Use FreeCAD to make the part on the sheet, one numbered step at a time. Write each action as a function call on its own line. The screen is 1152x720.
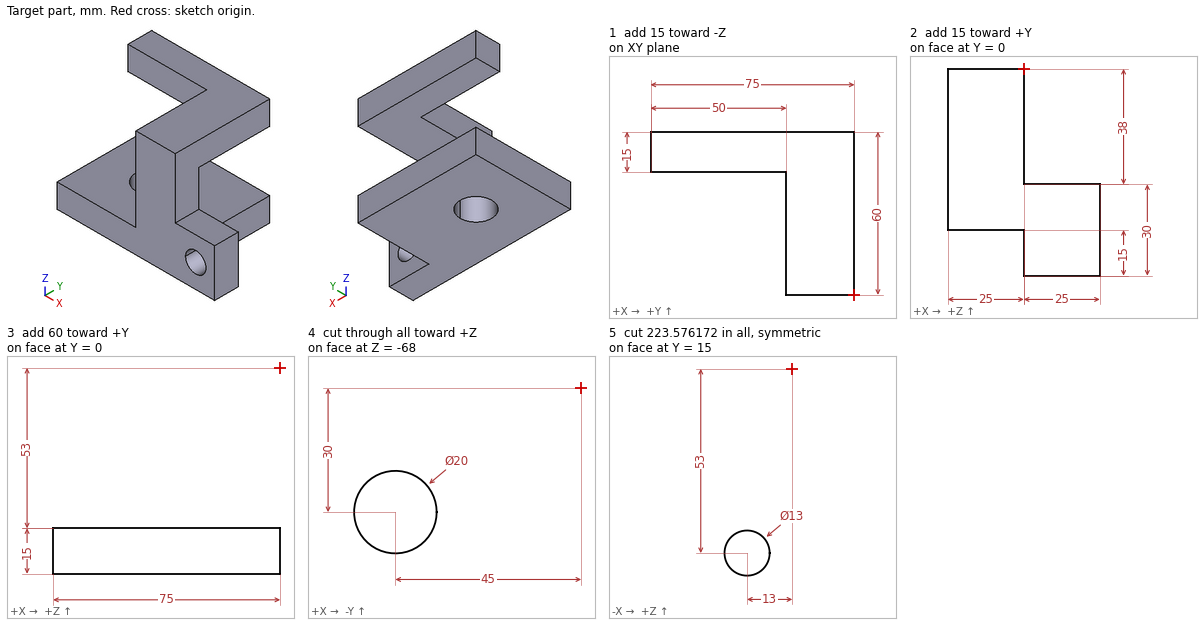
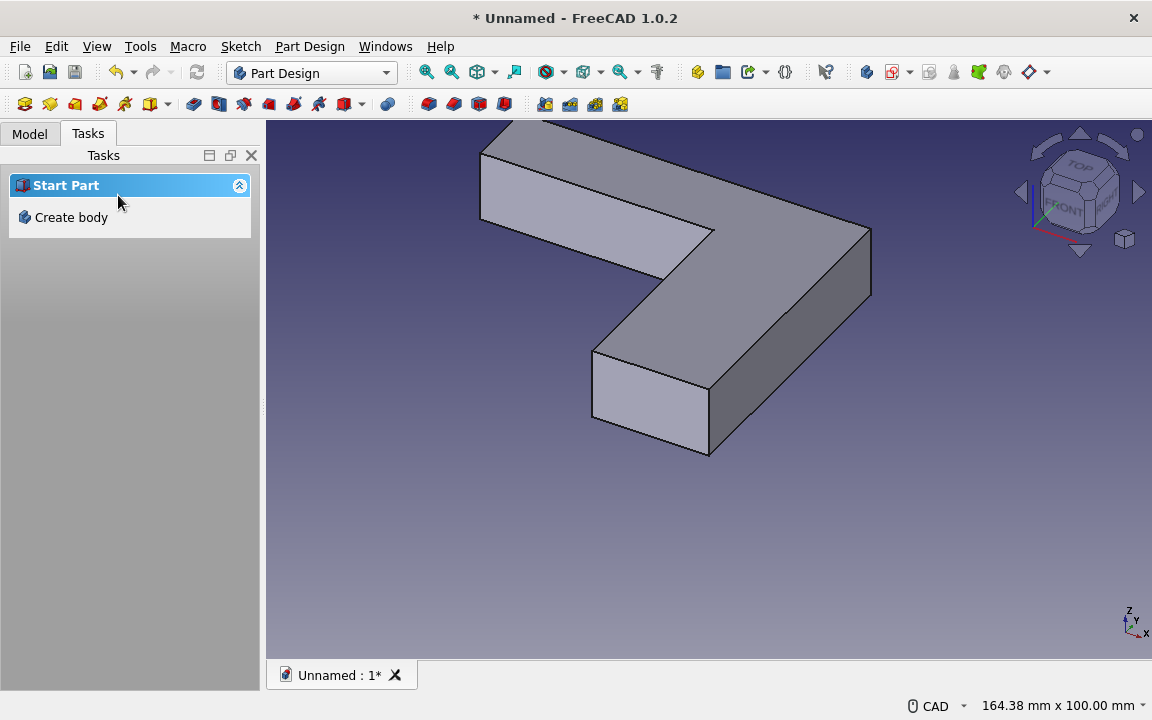
click(427, 72)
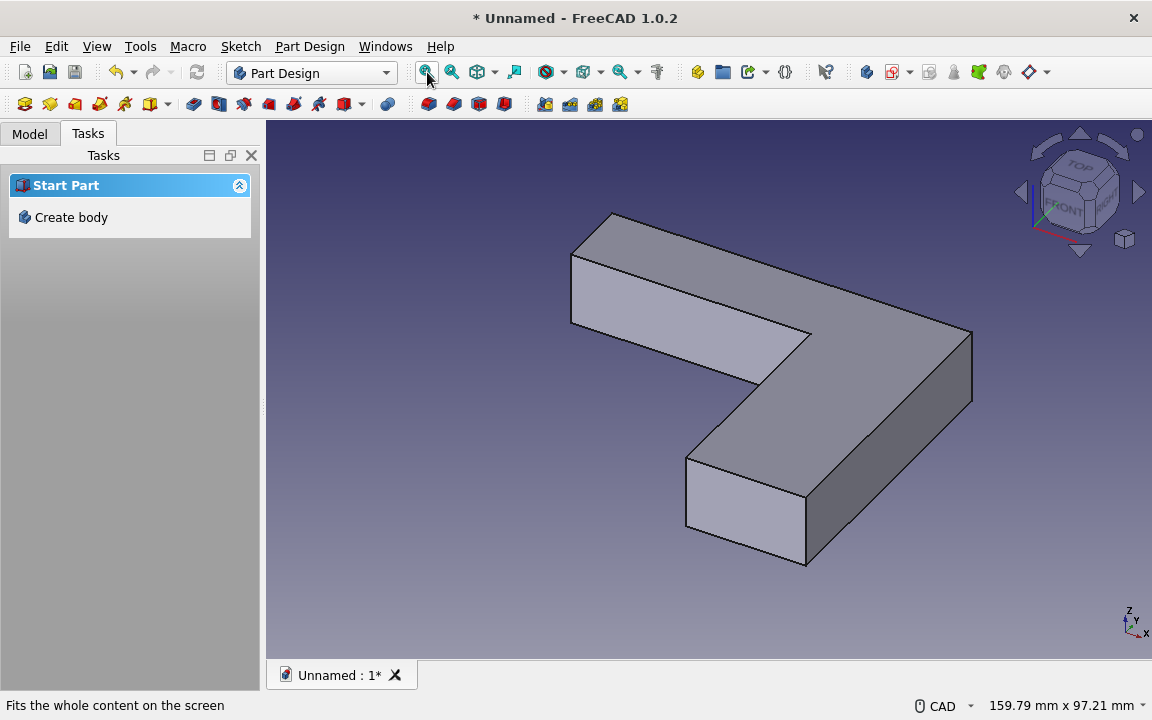
click(763, 517)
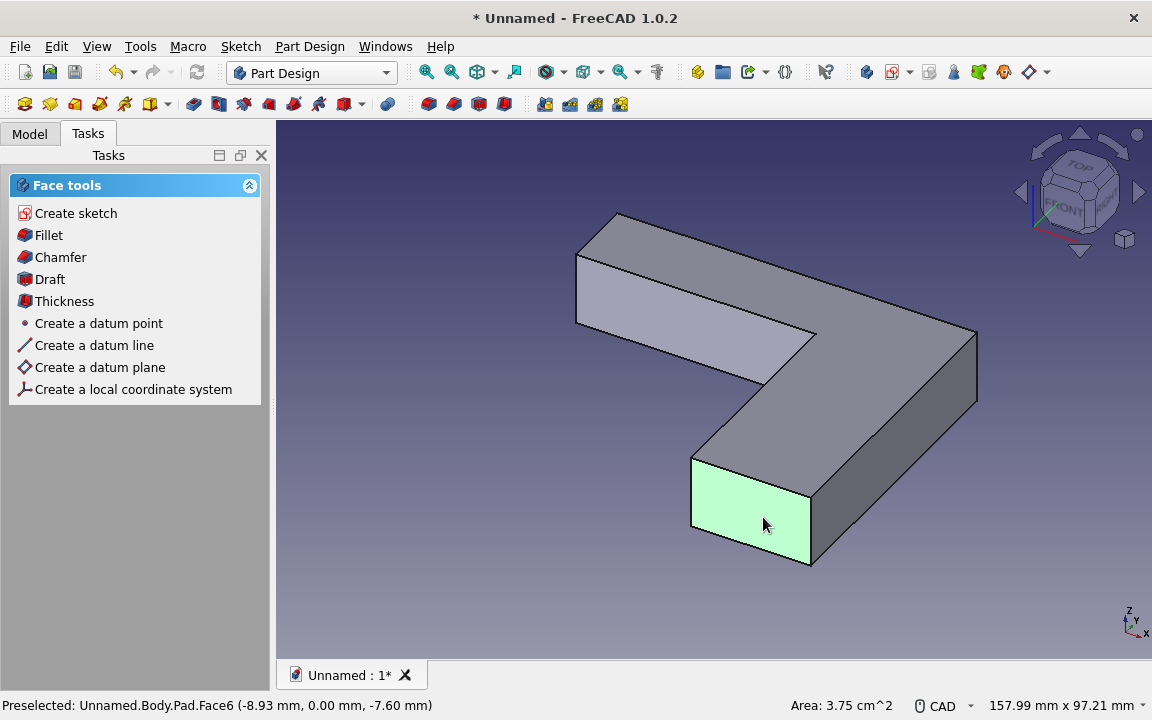
click(892, 72)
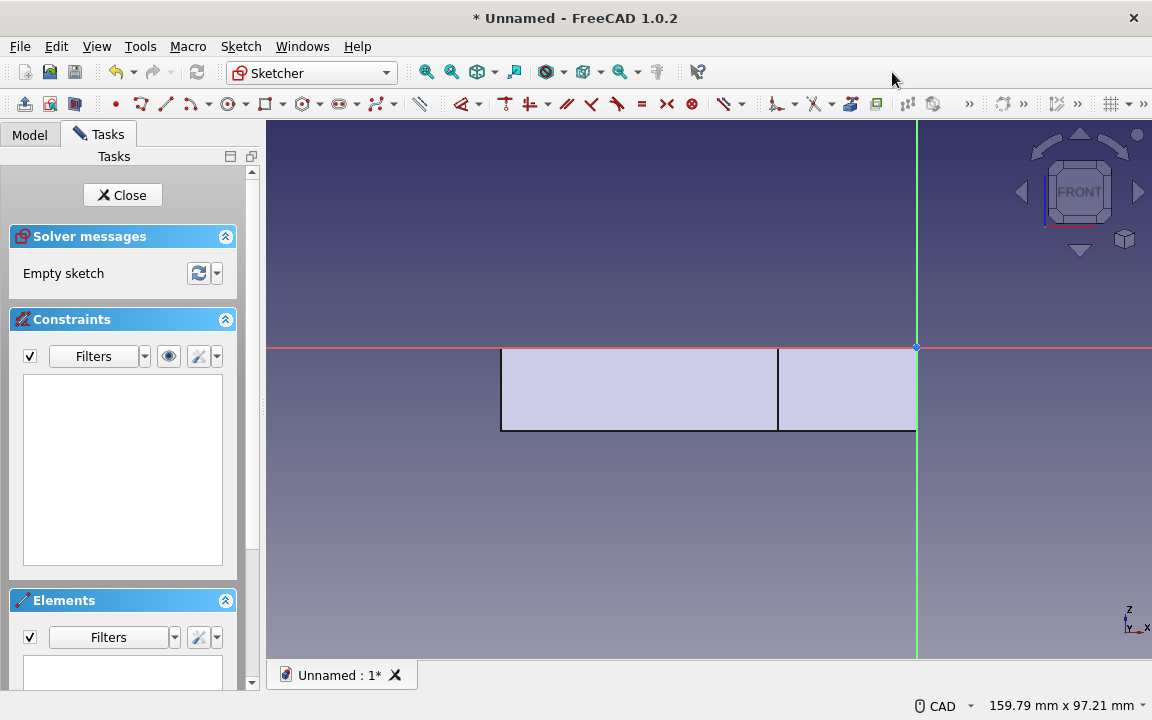
scroll(294, 148, down, 2)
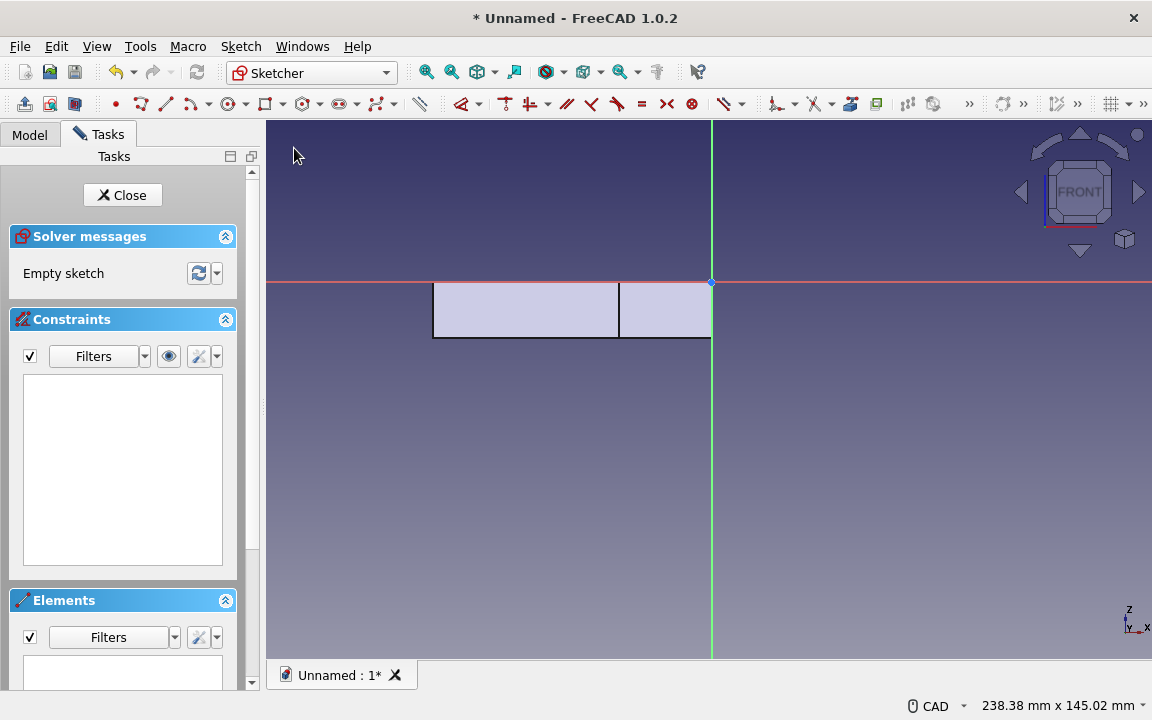
click(141, 104)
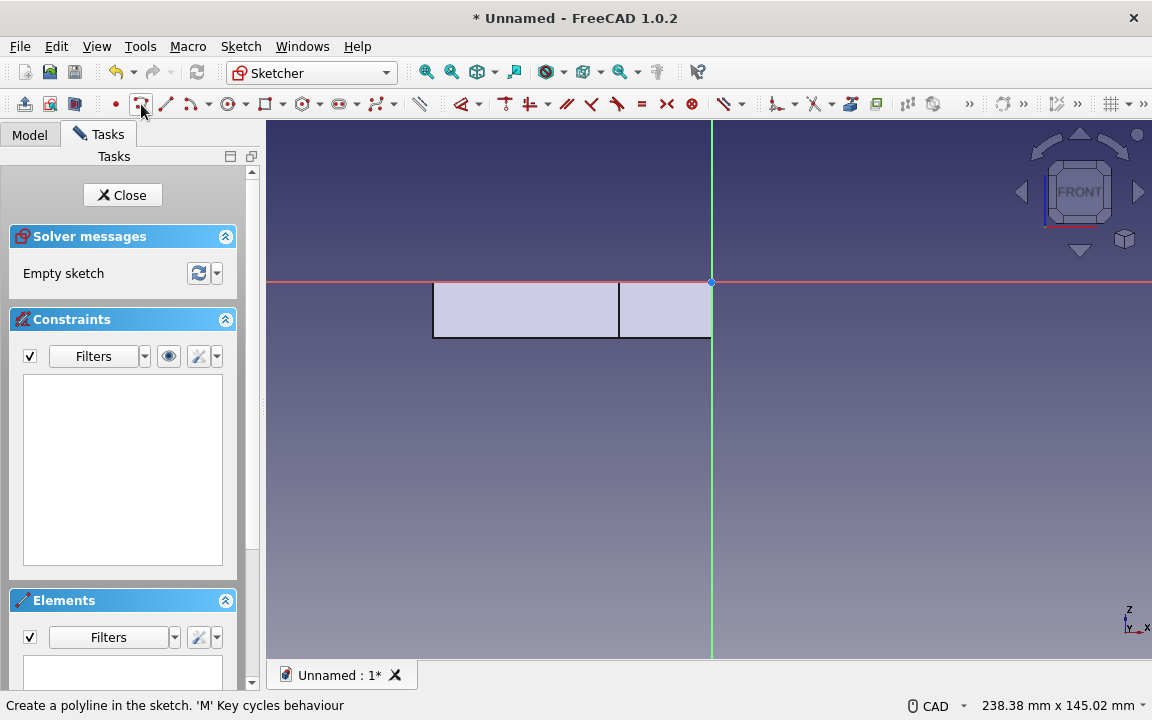
click(712, 282)
click(721, 423)
click(804, 423)
click(804, 535)
click(712, 535)
click(721, 479)
click(619, 479)
click(619, 291)
click(712, 282)
key(Escape)
key(Escape)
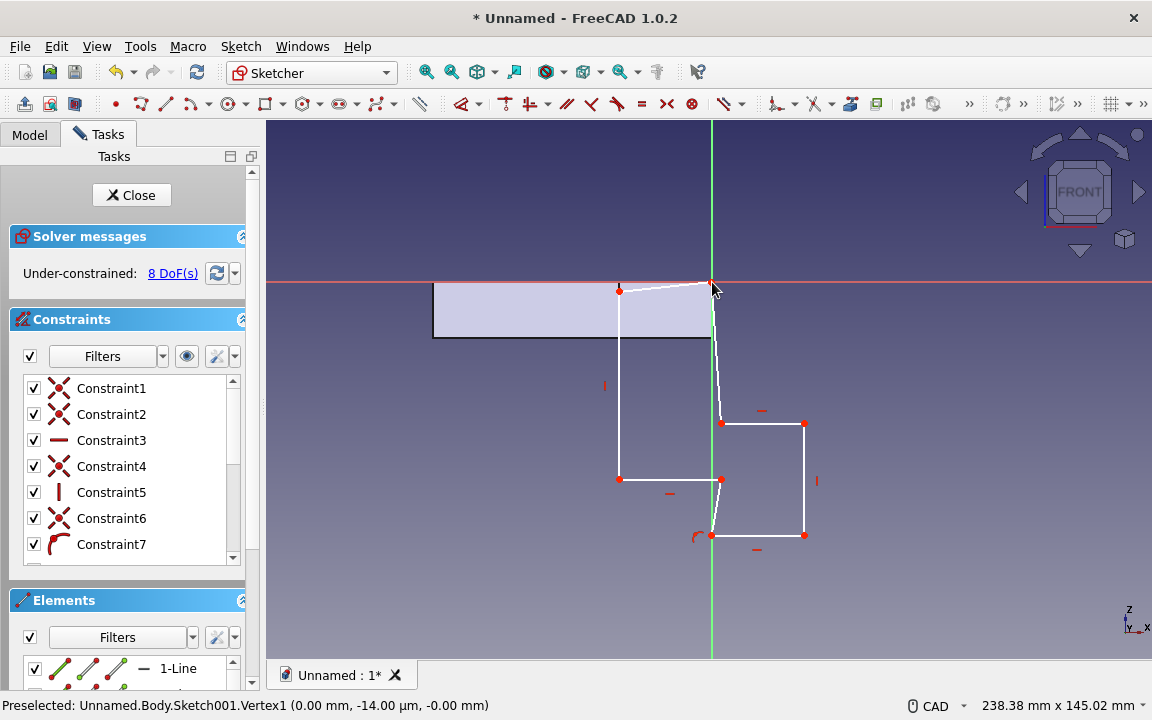
click(714, 325)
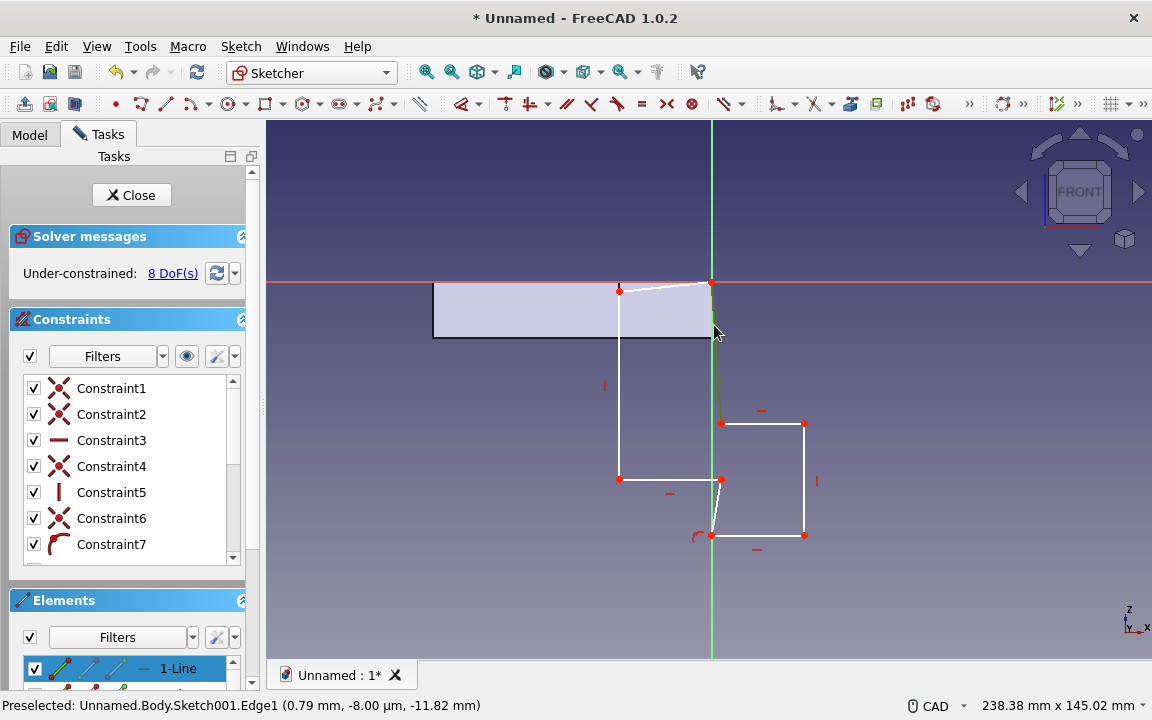
key(v)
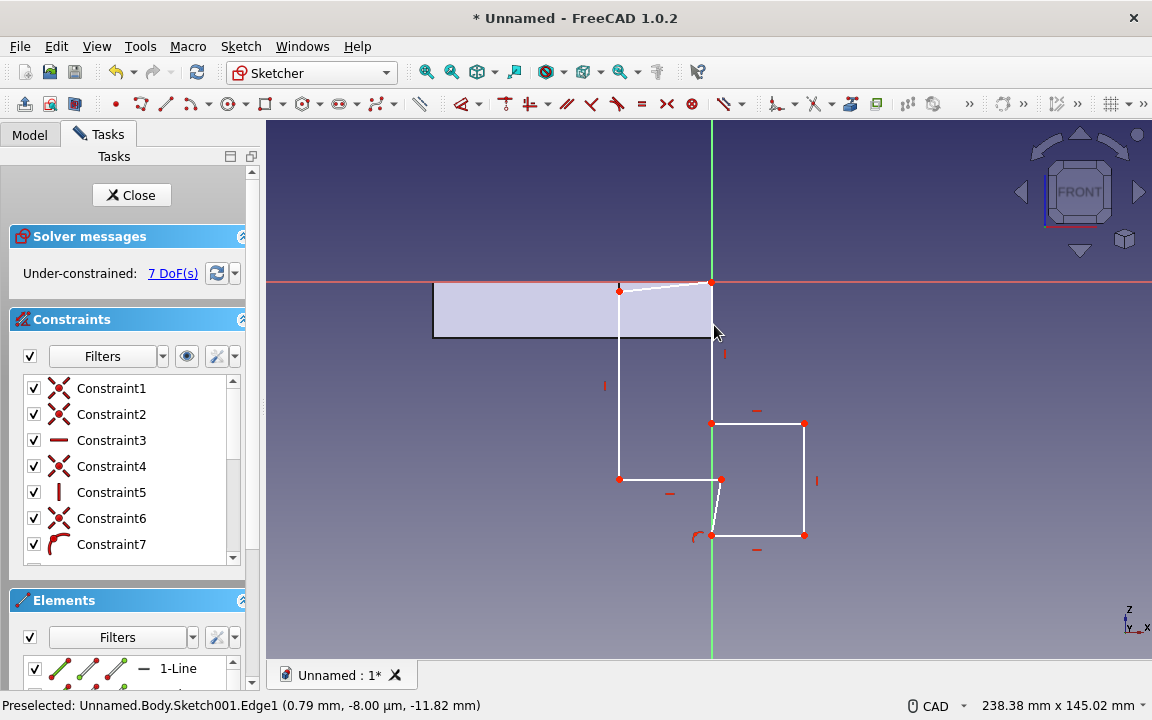
click(714, 519)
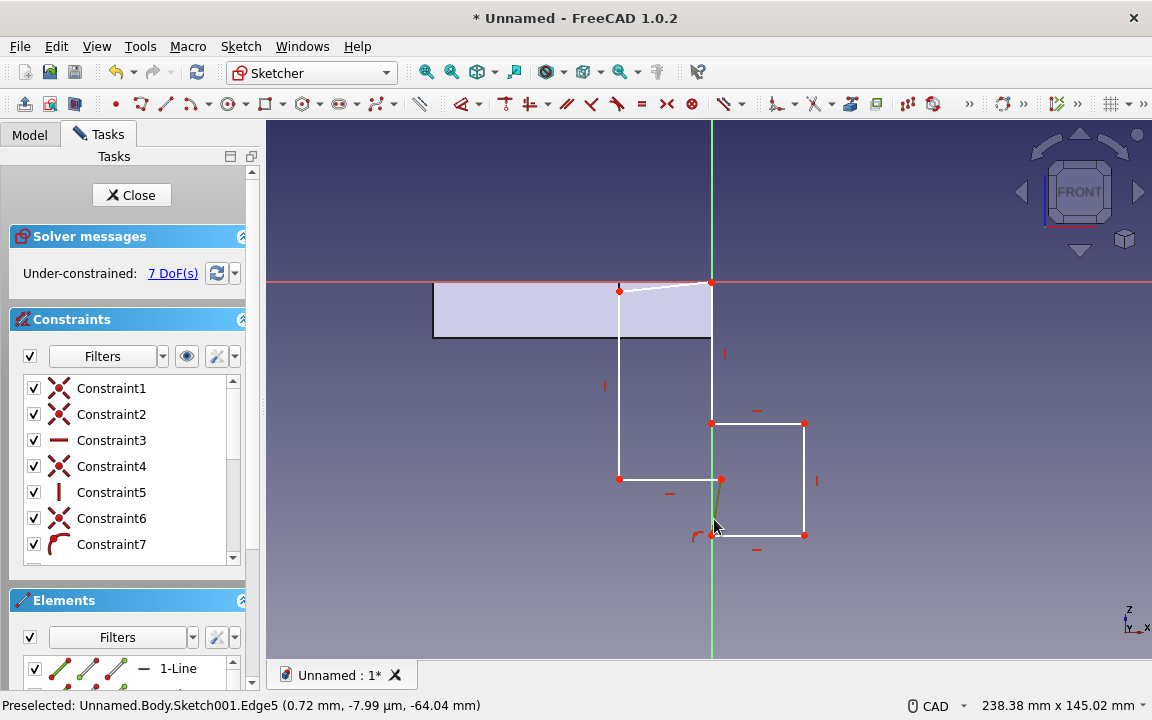
click(548, 104)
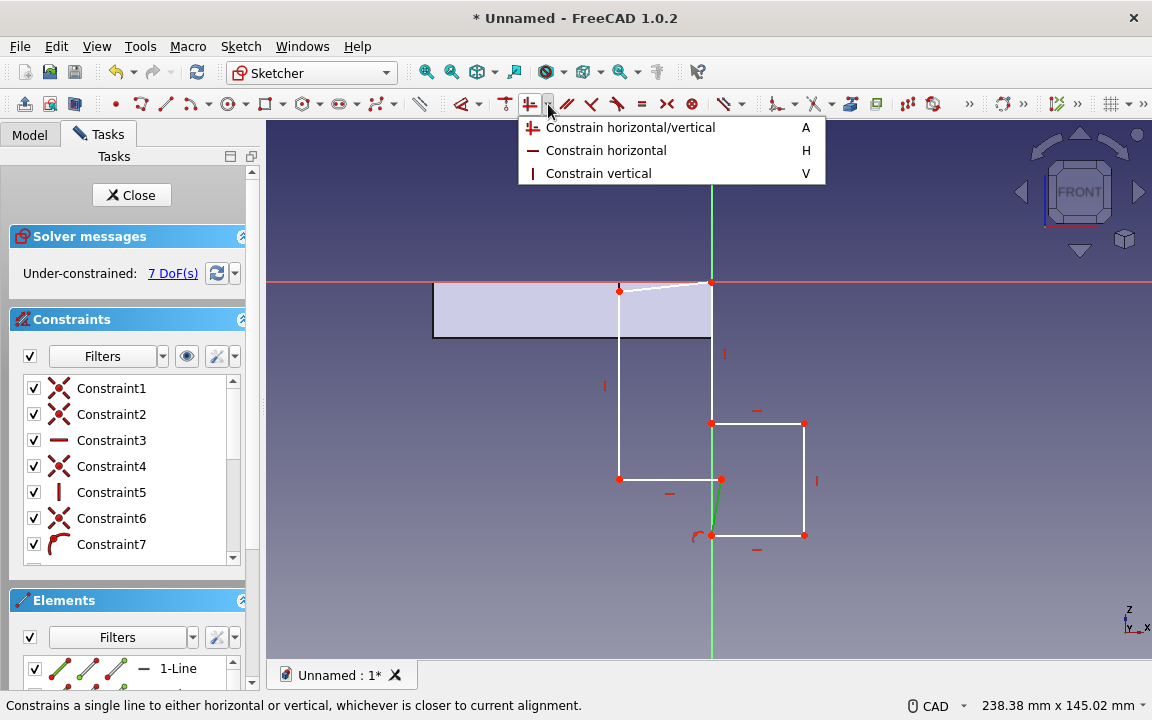
click(672, 174)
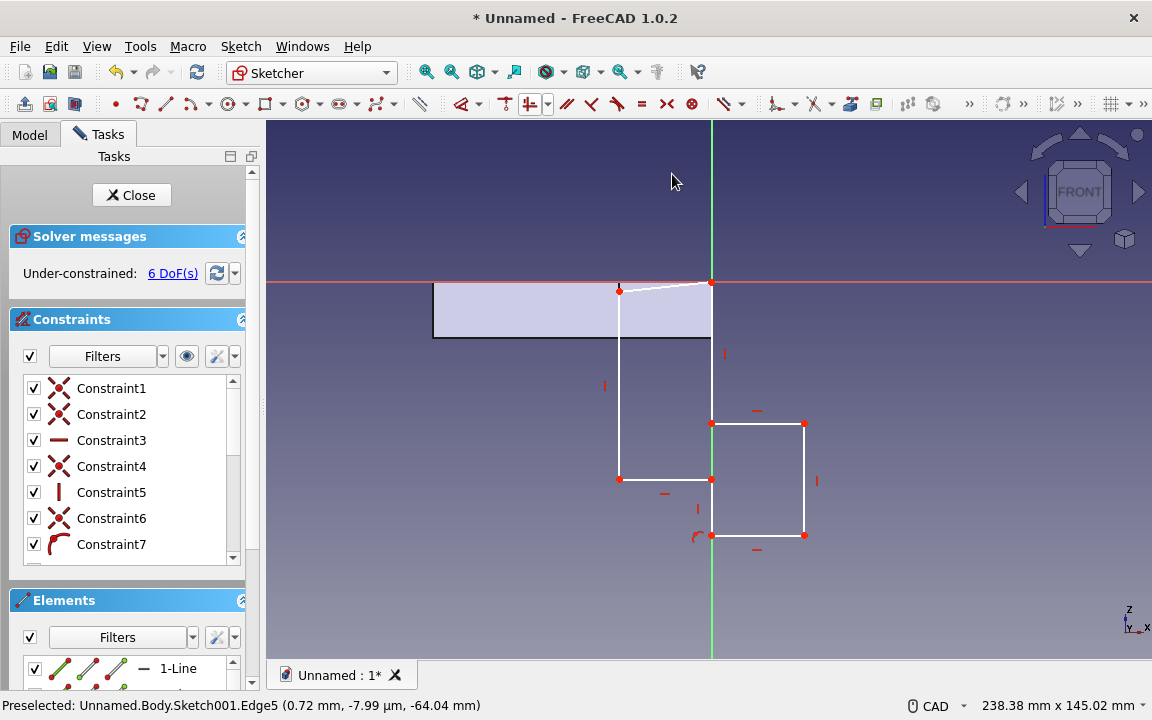
click(684, 285)